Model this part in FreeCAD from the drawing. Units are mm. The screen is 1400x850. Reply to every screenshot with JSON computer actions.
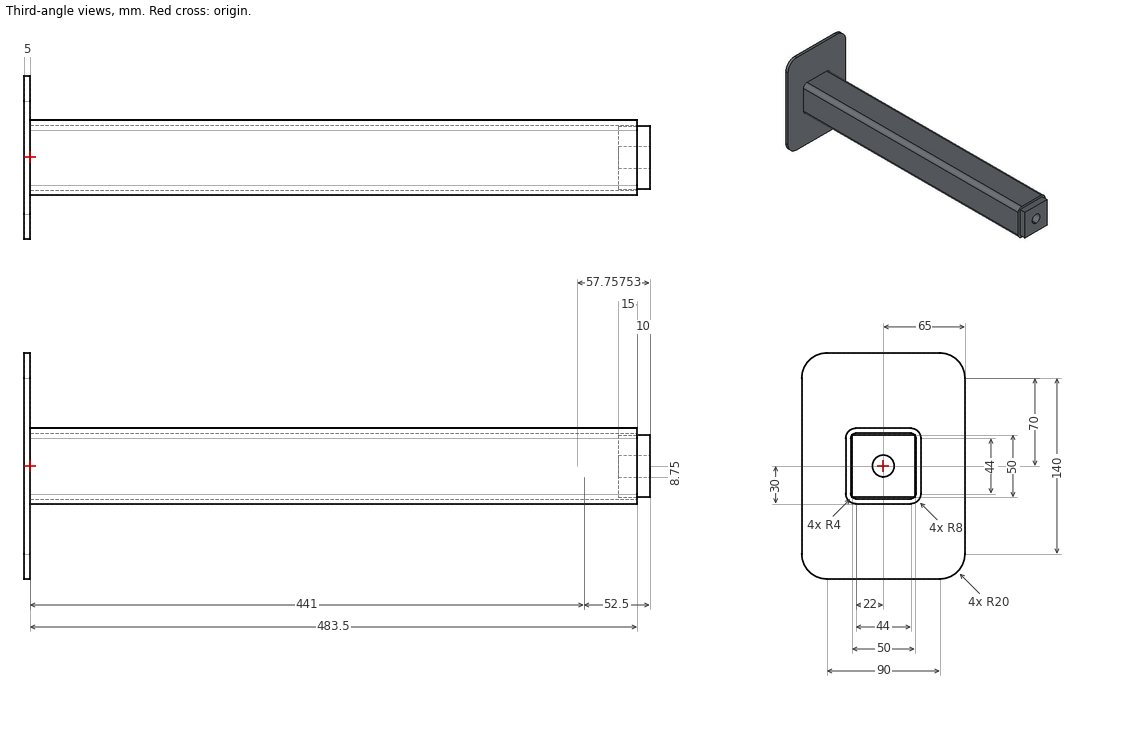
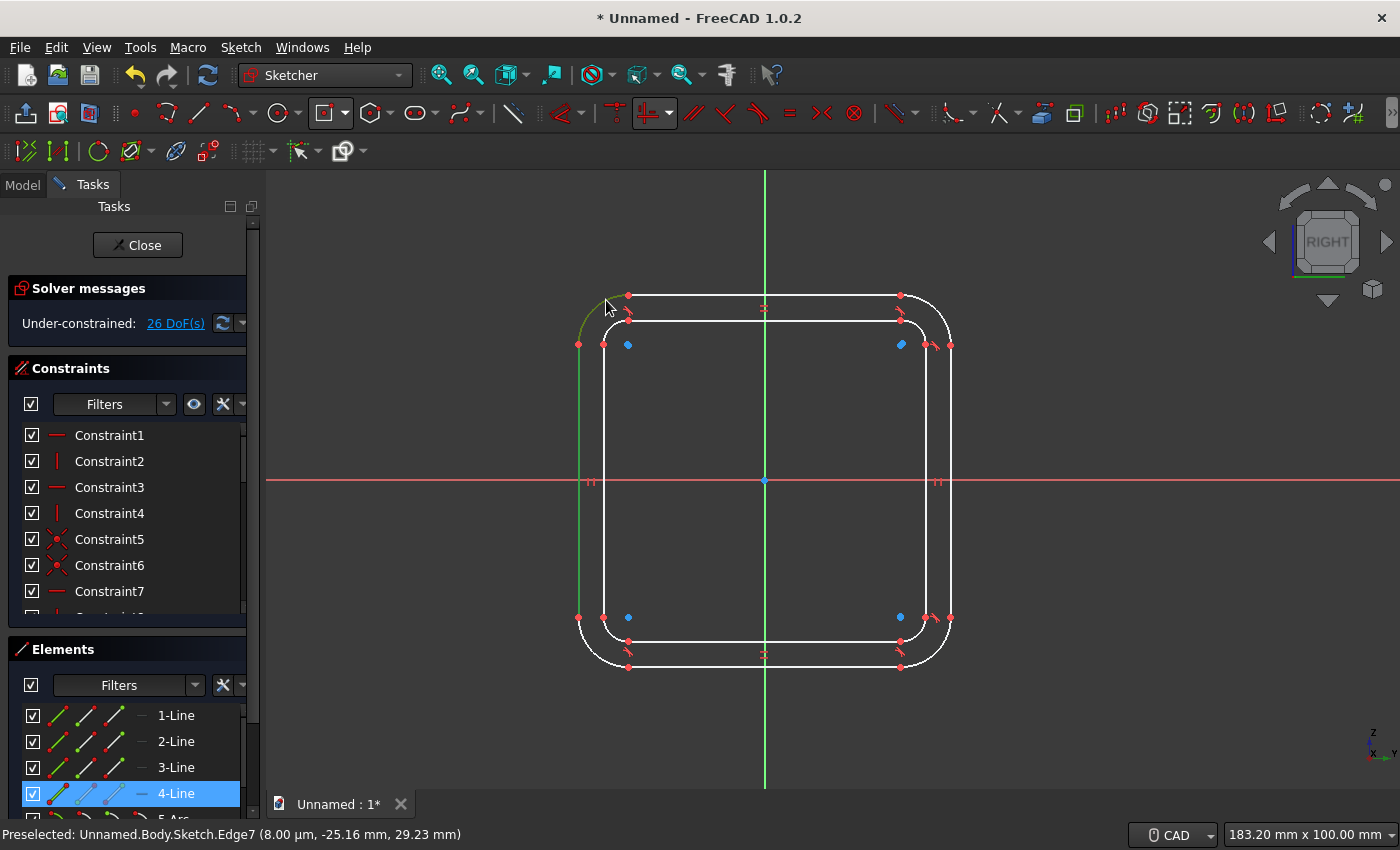
{"action": "left_click", "coordinate": [758, 114]}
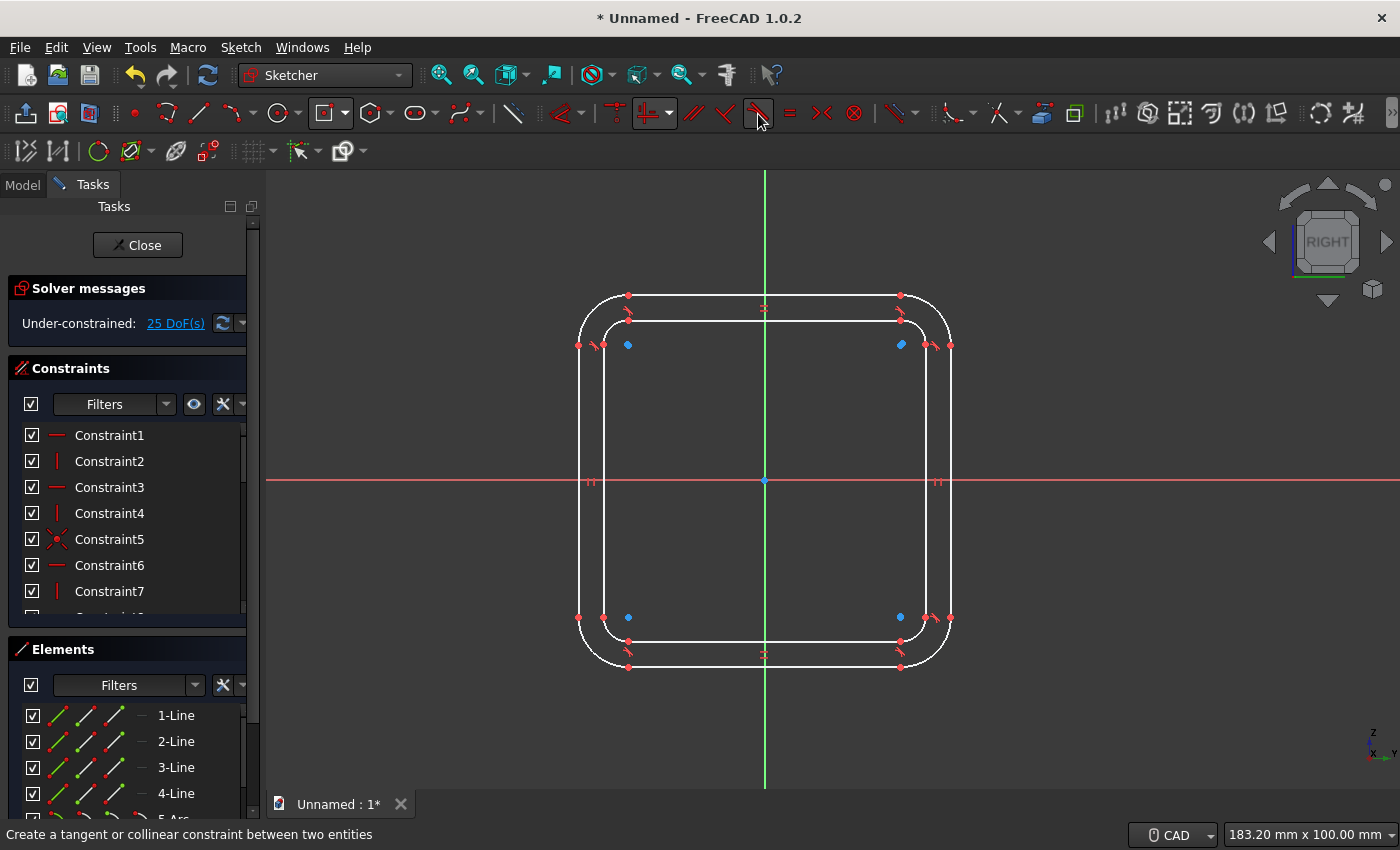
{"action": "left_click", "coordinate": [579, 427]}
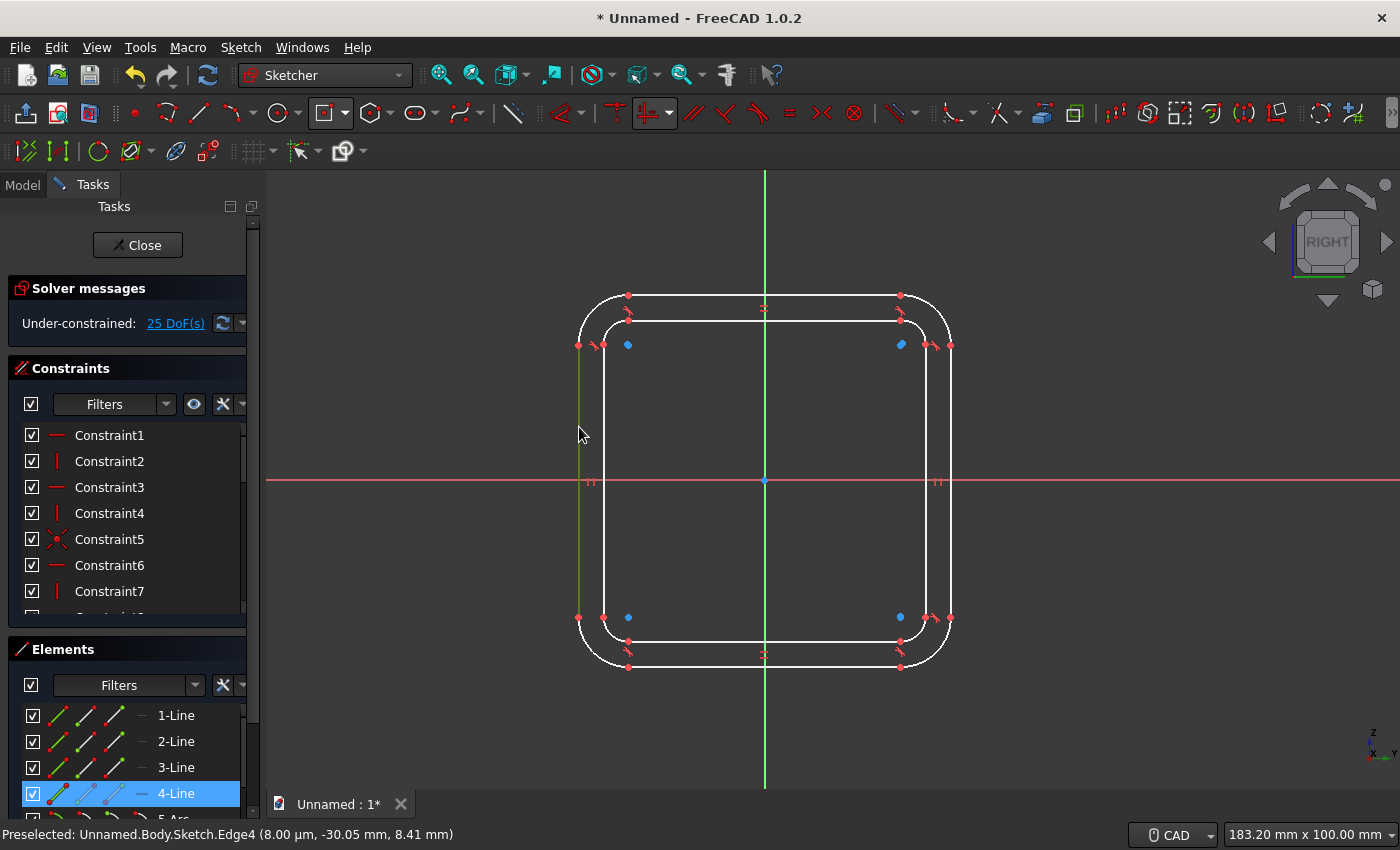
{"action": "left_click", "coordinate": [584, 640]}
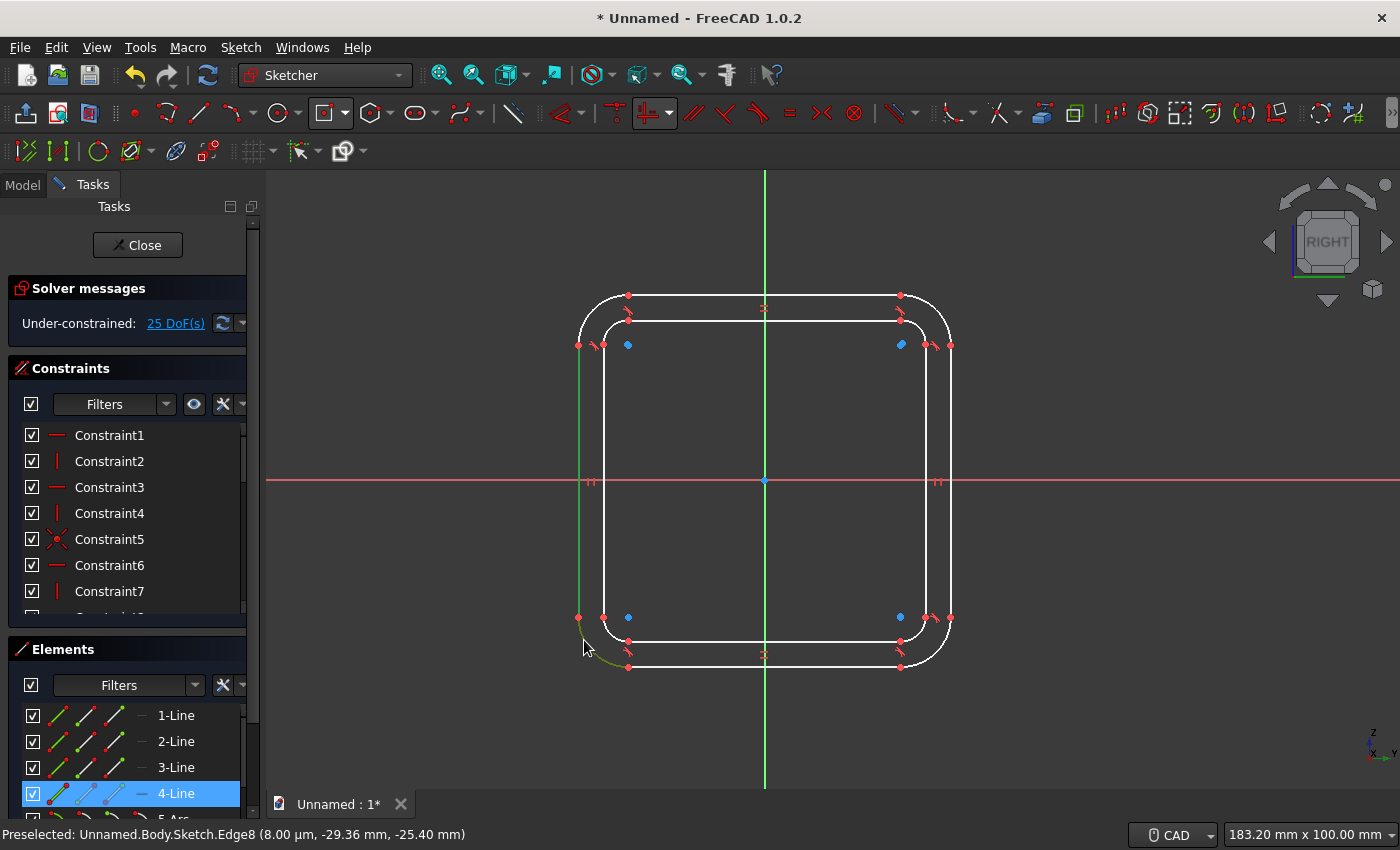
{"action": "key", "text": "t"}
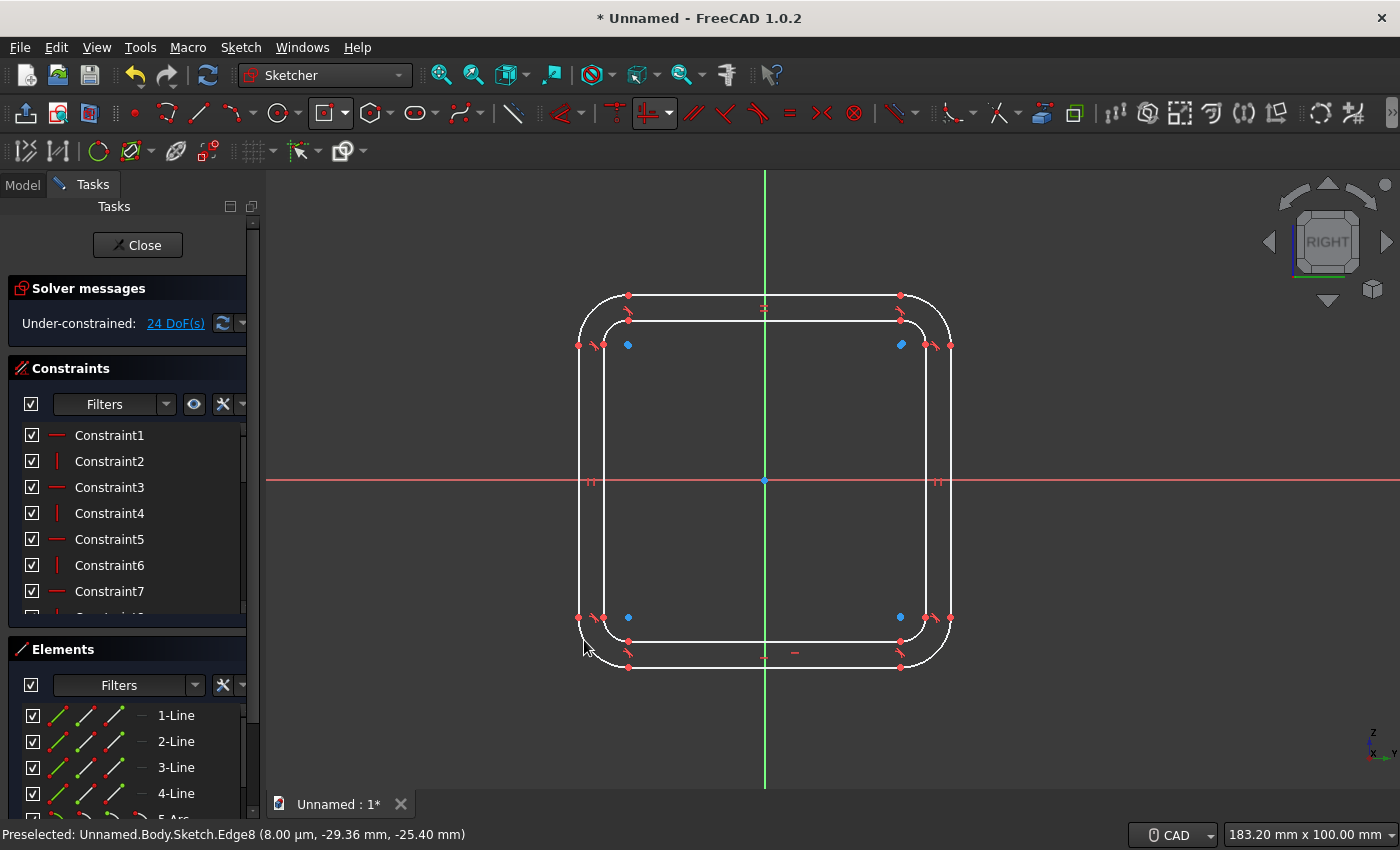
{"action": "left_click", "coordinate": [819, 642]}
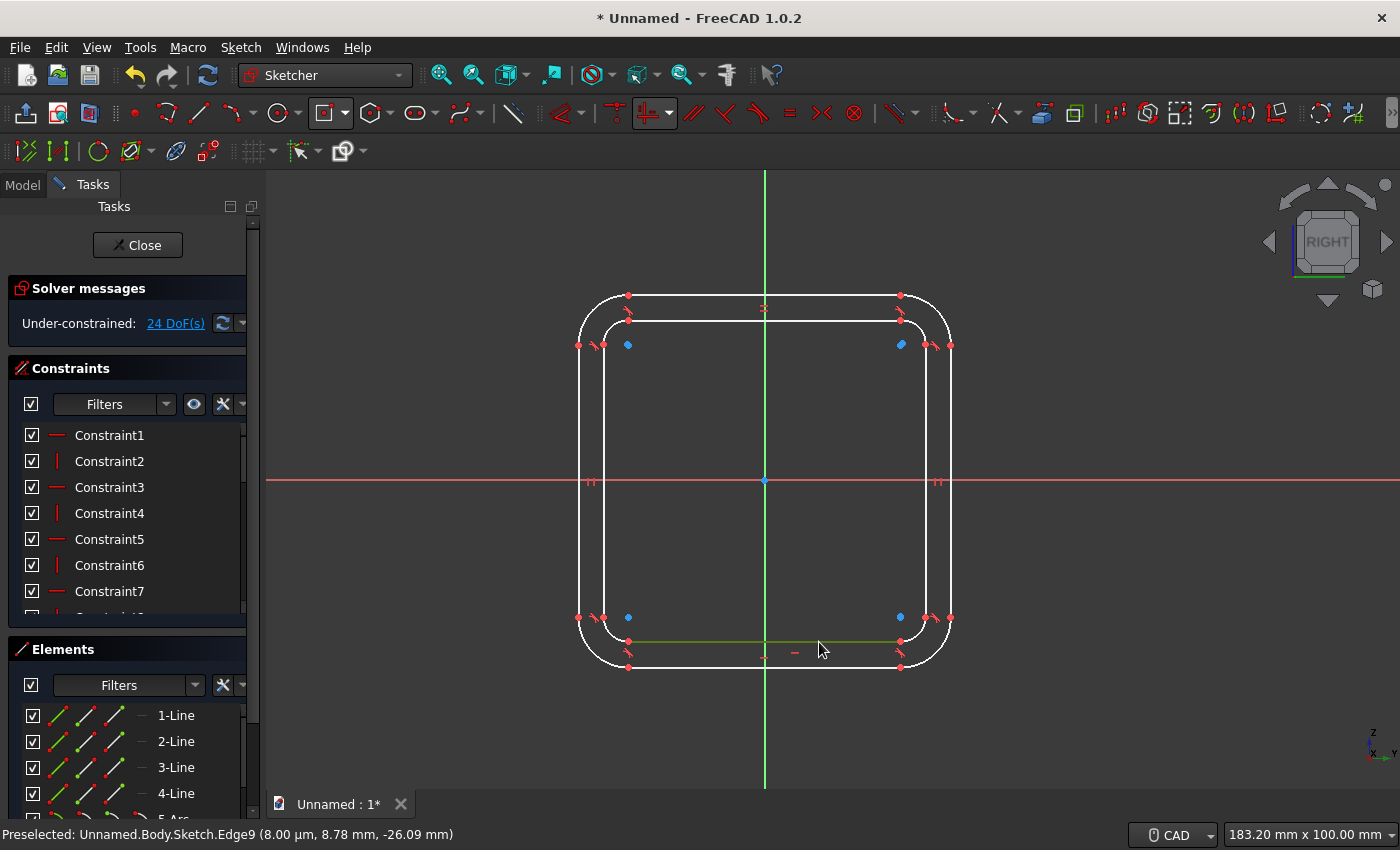
{"action": "left_click", "coordinate": [607, 629]}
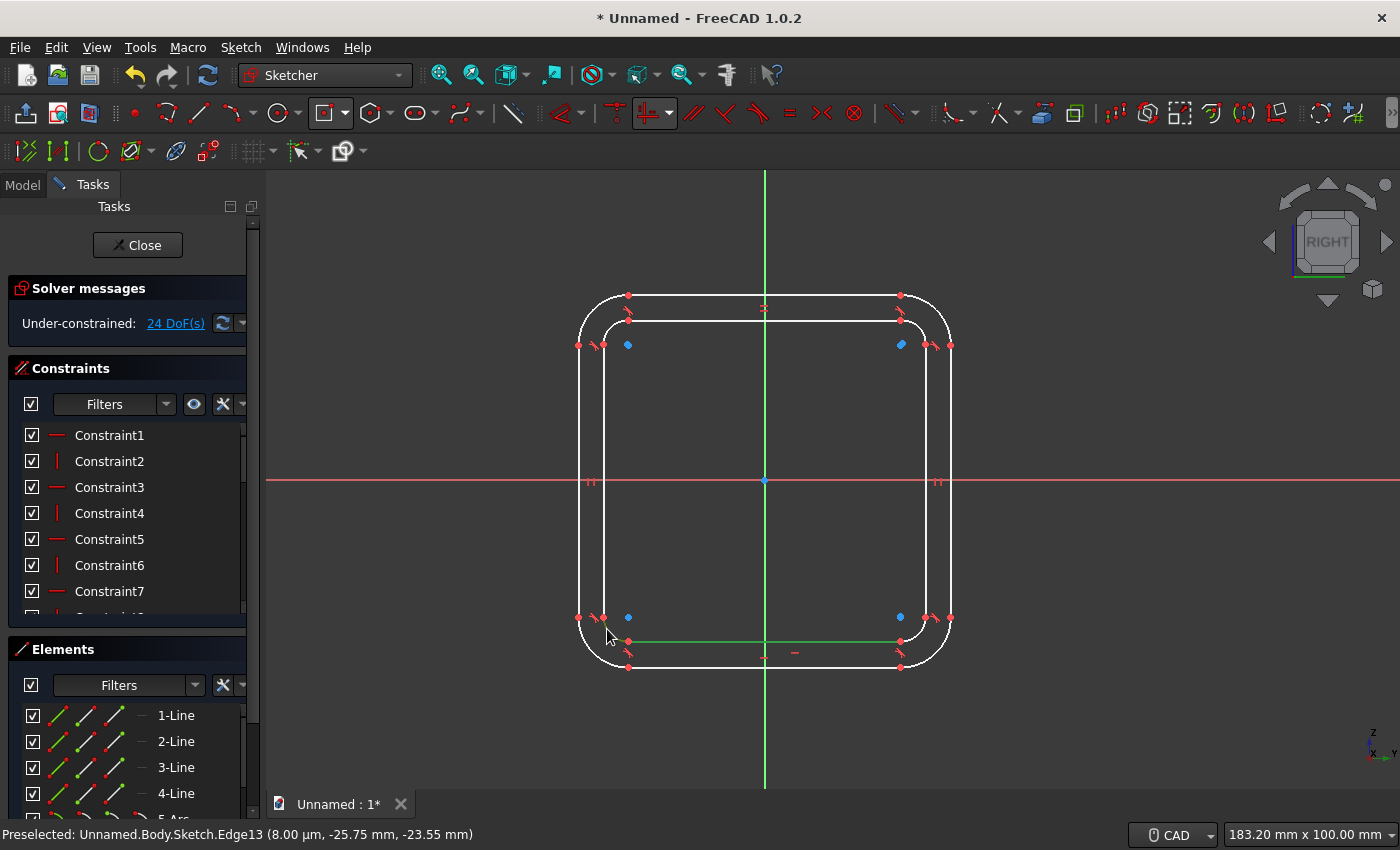
{"action": "key", "text": "t"}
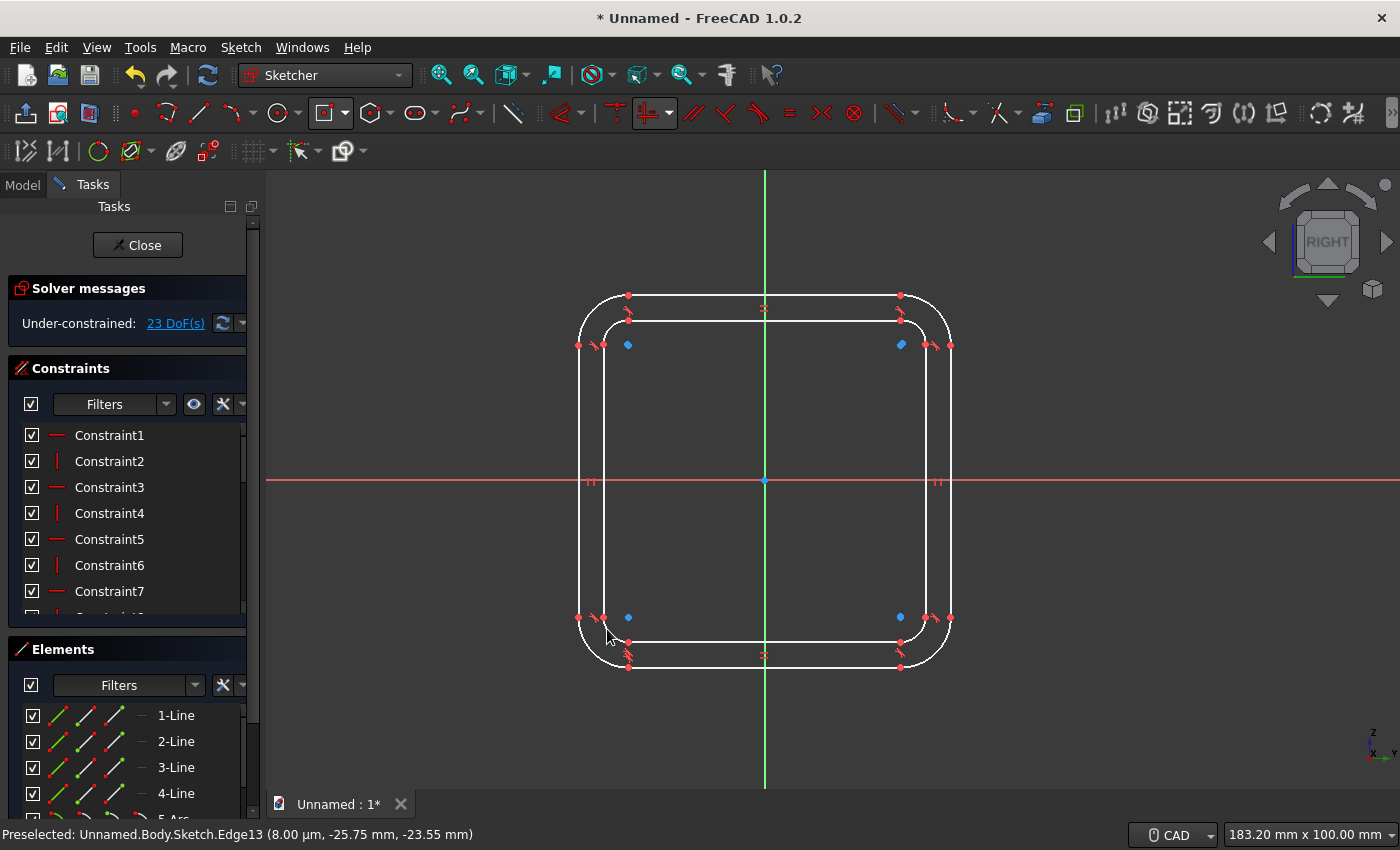
{"action": "left_click", "coordinate": [819, 642]}